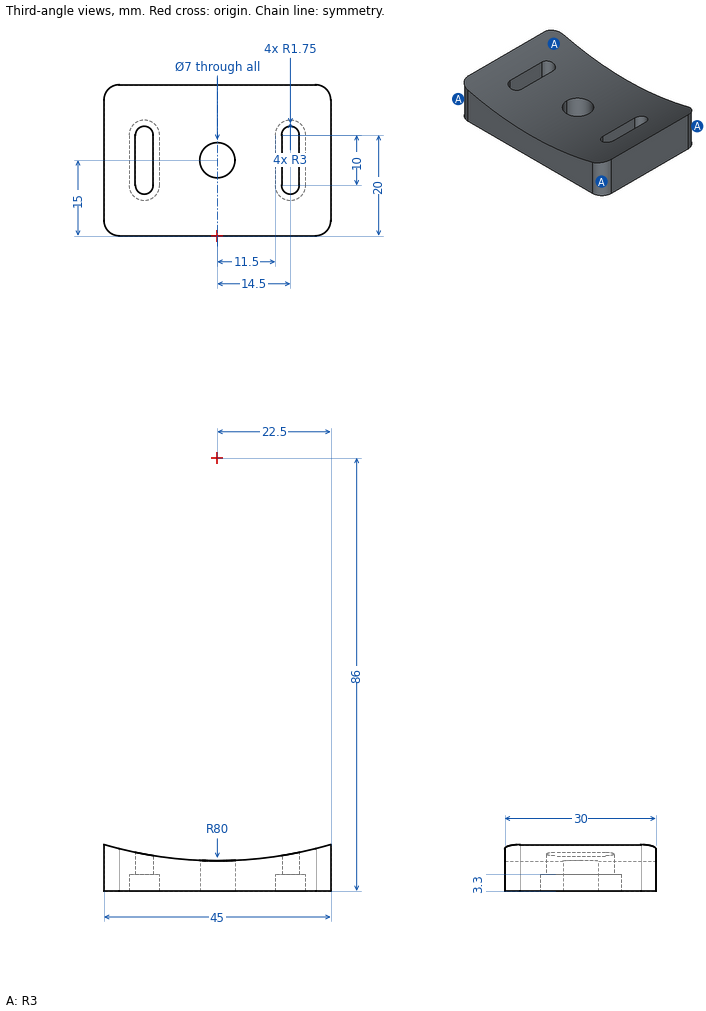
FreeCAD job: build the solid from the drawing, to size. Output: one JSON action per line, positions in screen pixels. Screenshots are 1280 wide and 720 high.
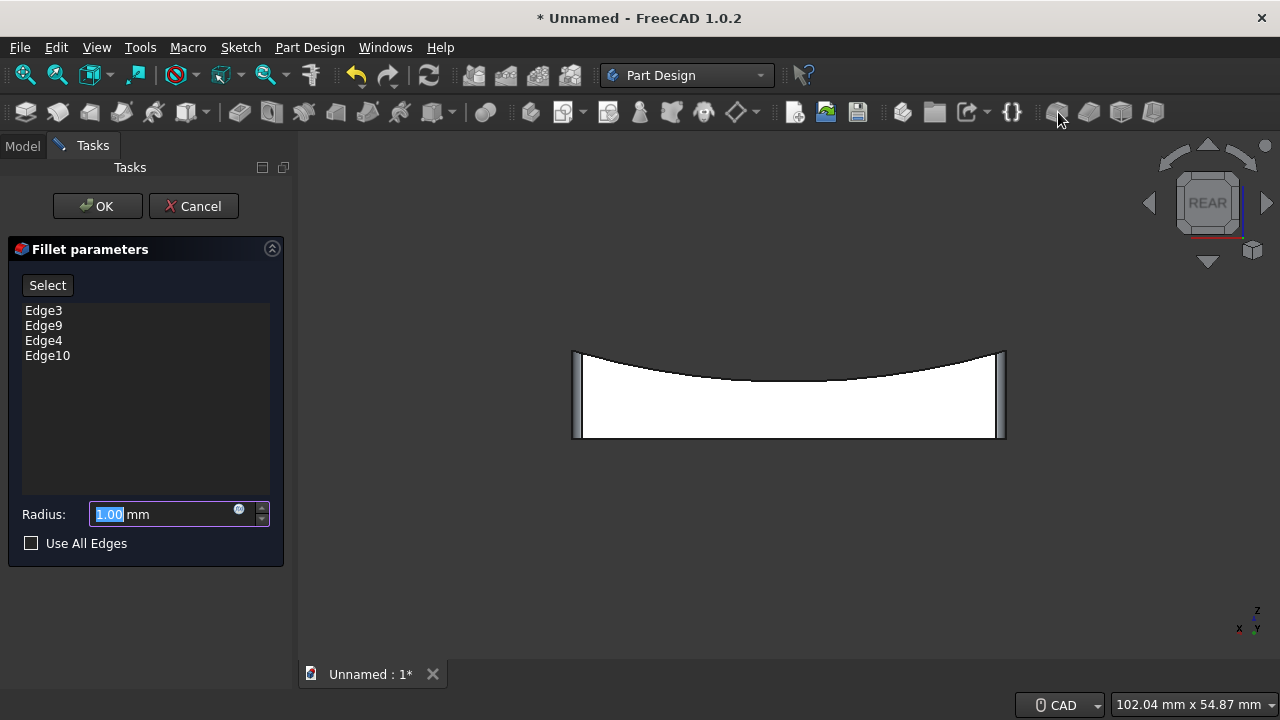
{"action": "type", "text": "3"}
{"action": "key", "text": "Tab"}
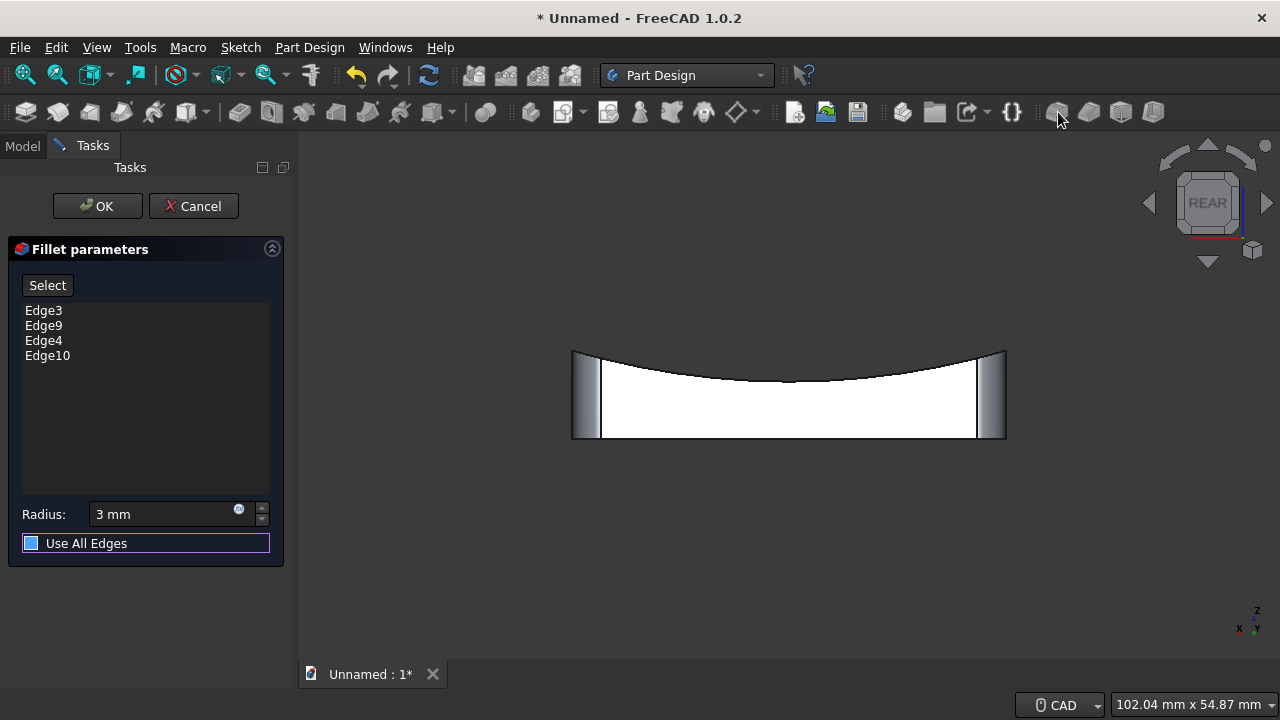
{"action": "left_click", "coordinate": [98, 206]}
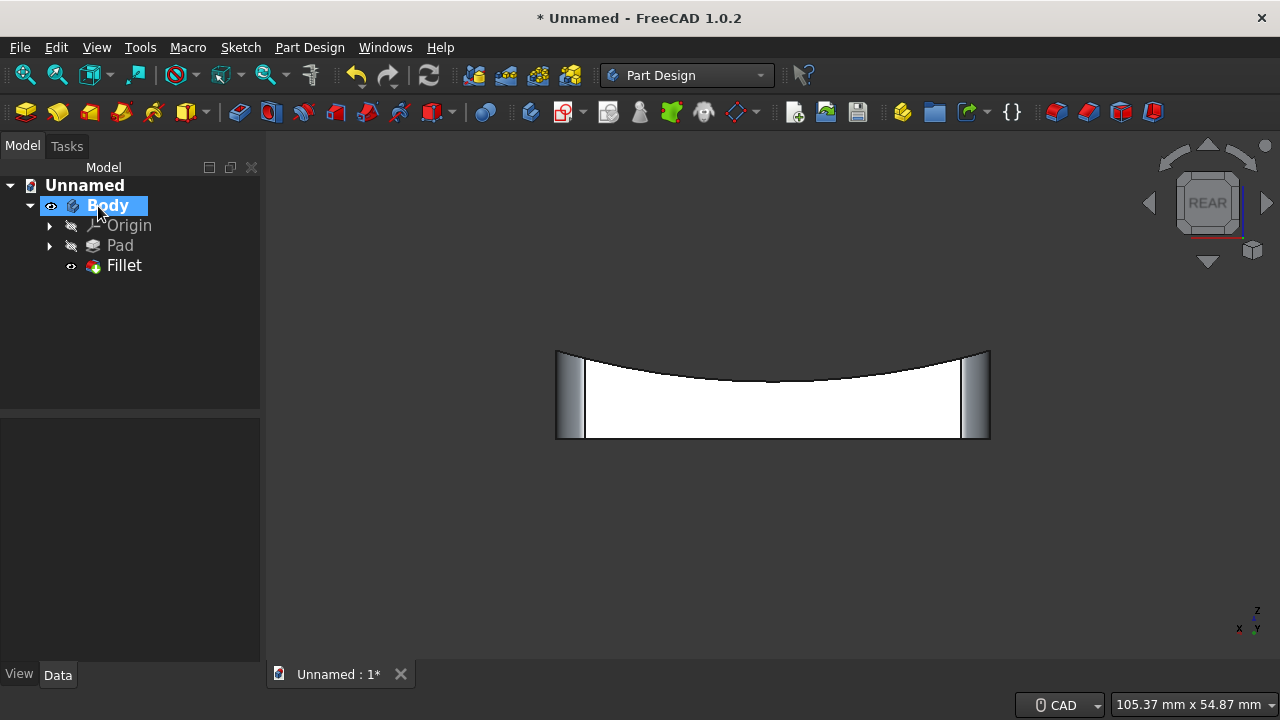
{"action": "key", "text": "v f"}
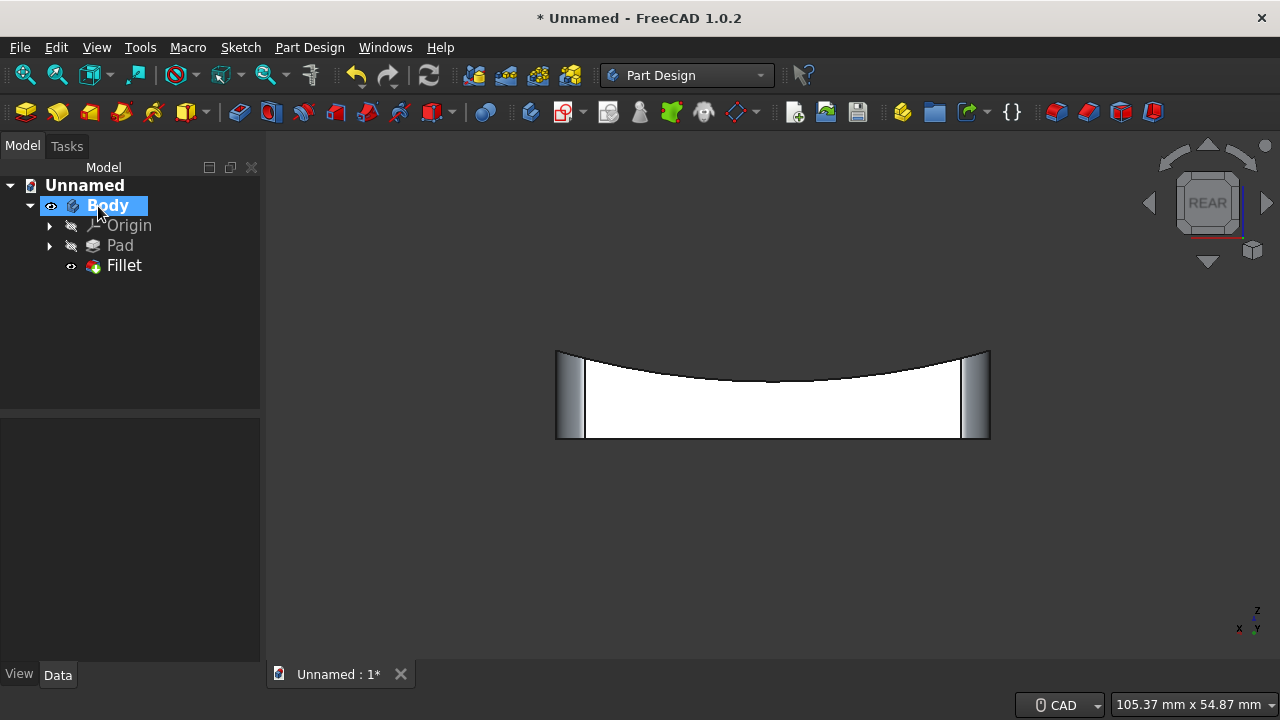
{"action": "key", "text": "5"}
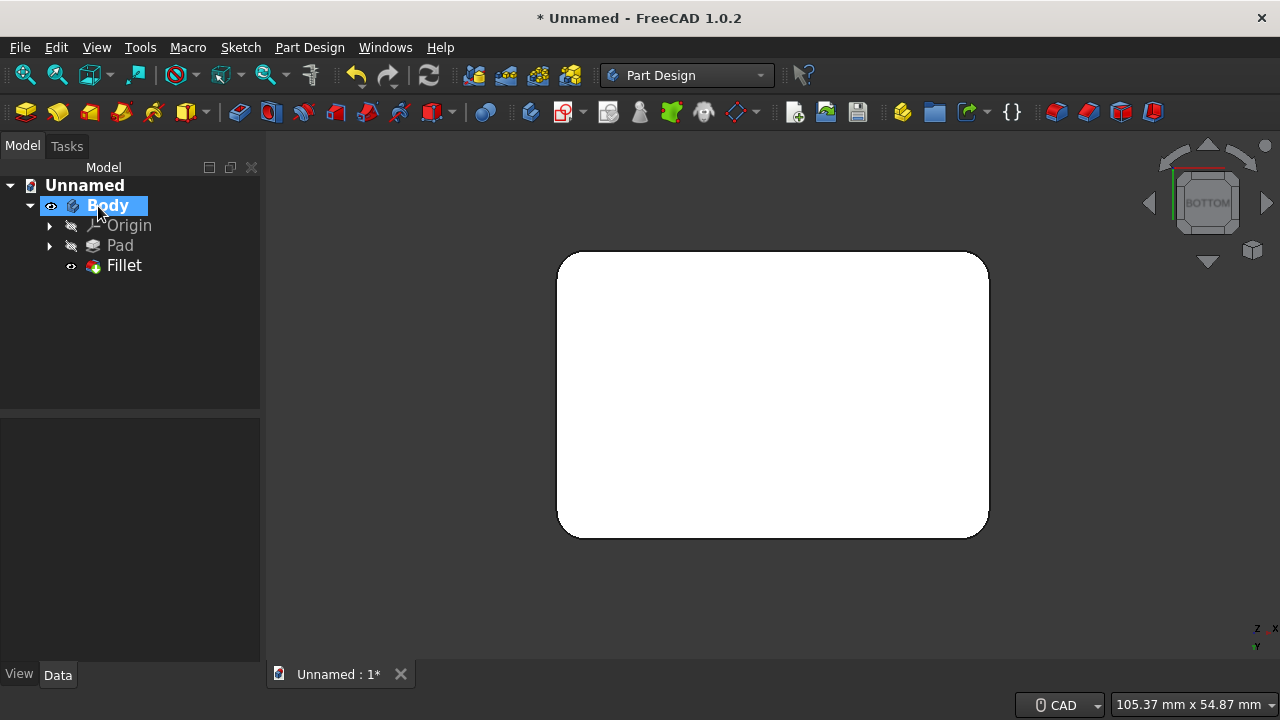
{"action": "left_click", "coordinate": [835, 394]}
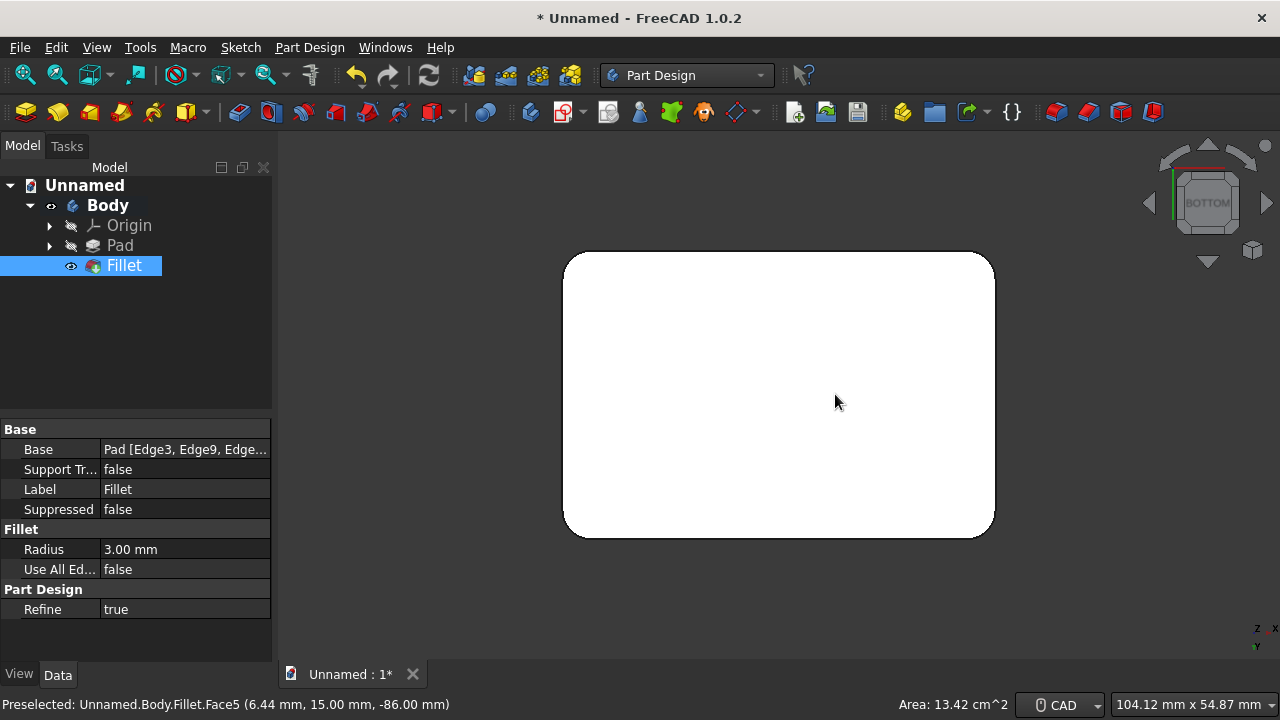
{"action": "left_click", "coordinate": [564, 112]}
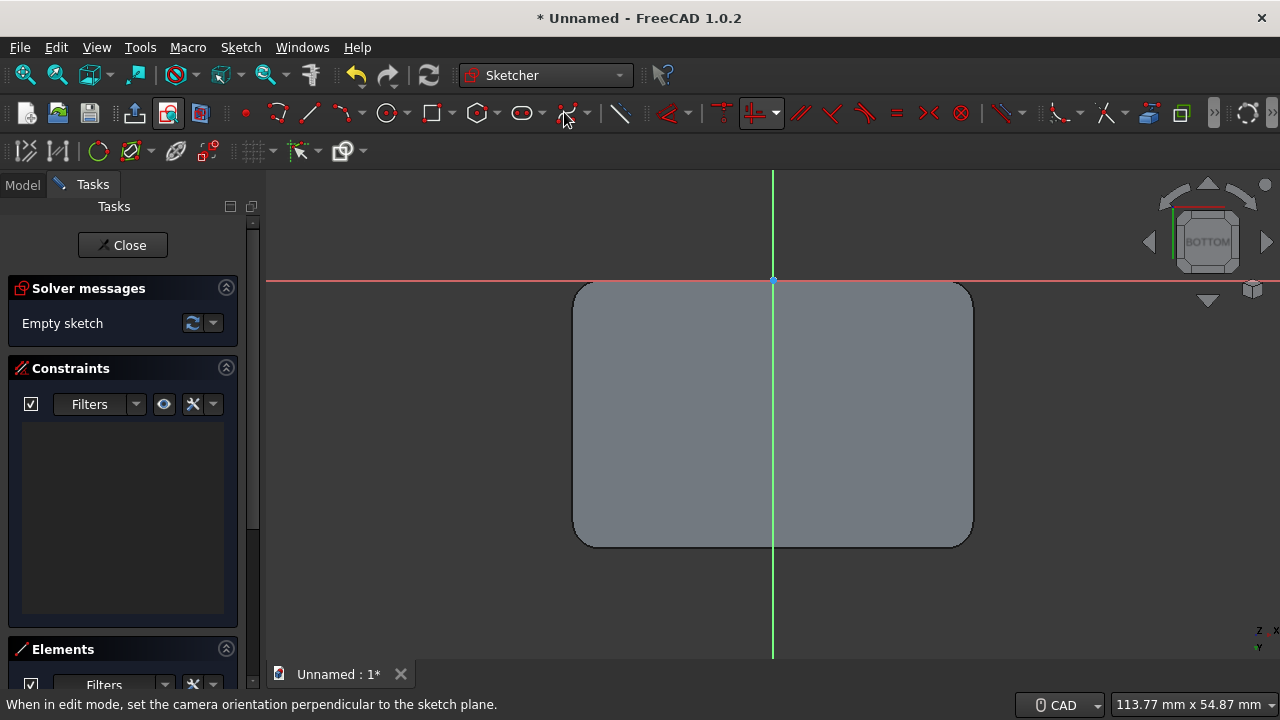
{"action": "scroll", "coordinate": [790, 414], "scroll_direction": "up", "scroll_amount": 8}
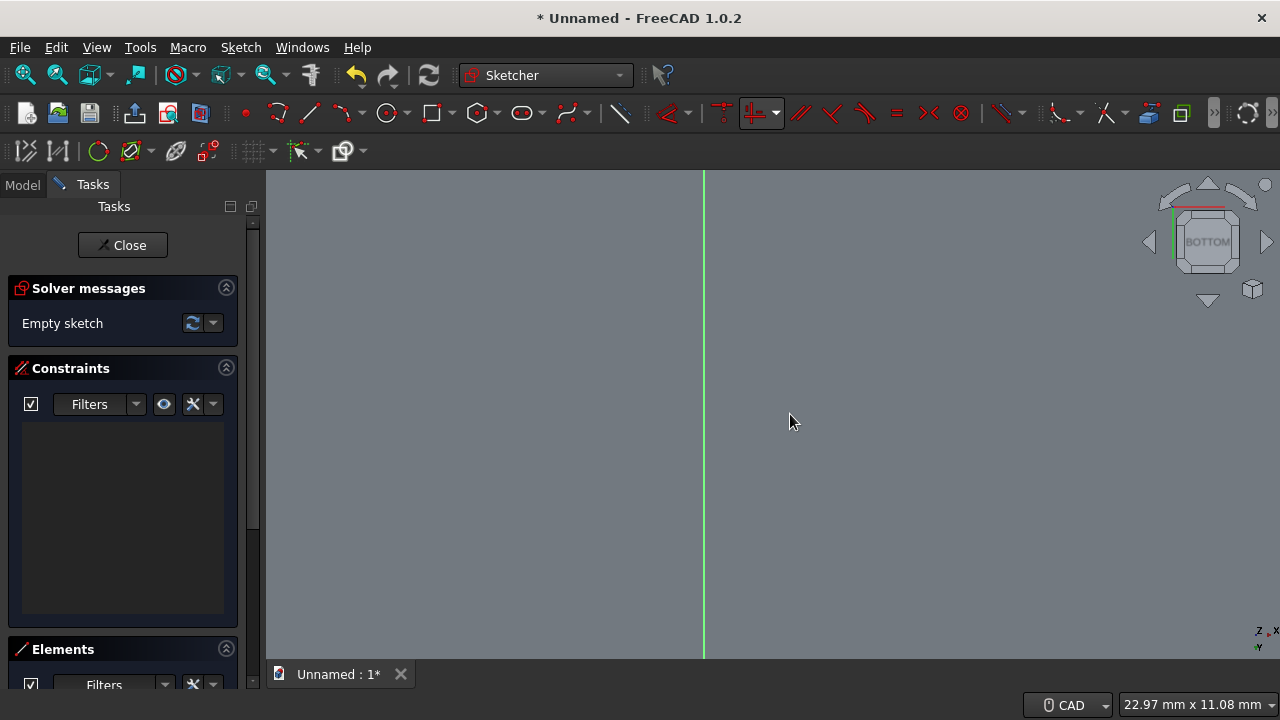
{"action": "left_click", "coordinate": [388, 114]}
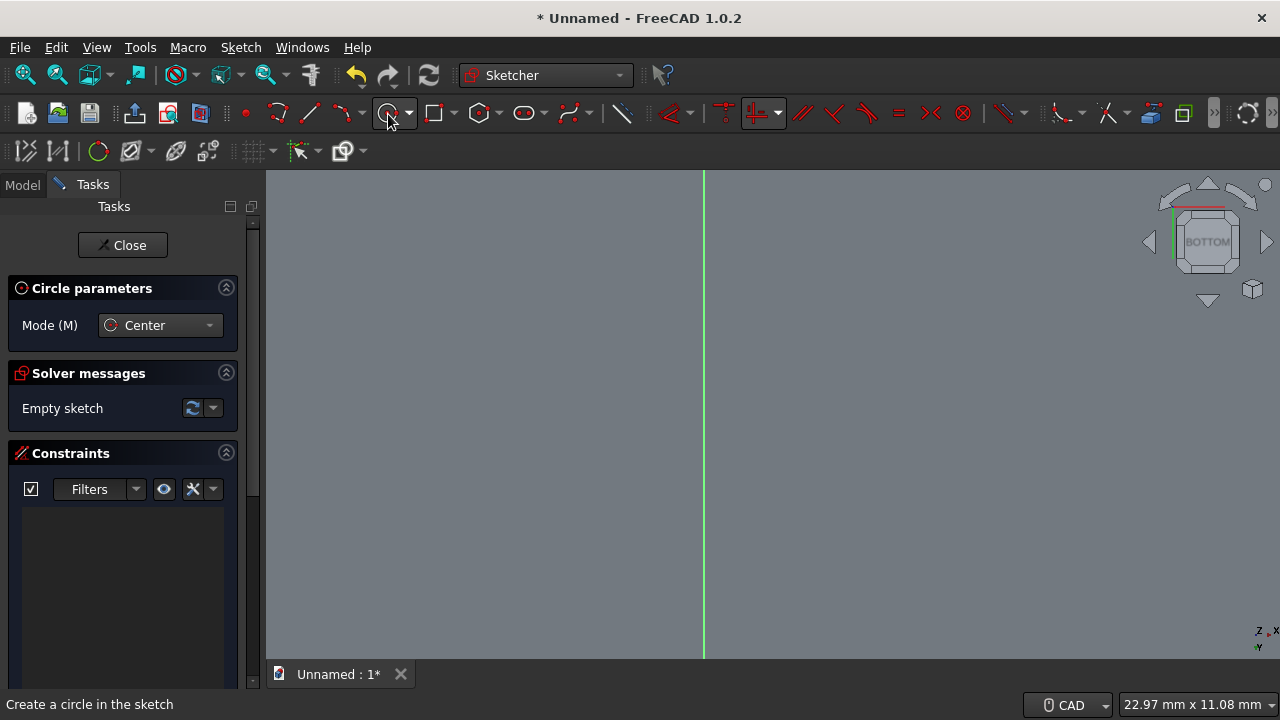
{"action": "left_click", "coordinate": [704, 414]}
{"action": "mouse_move", "coordinate": [813, 305]}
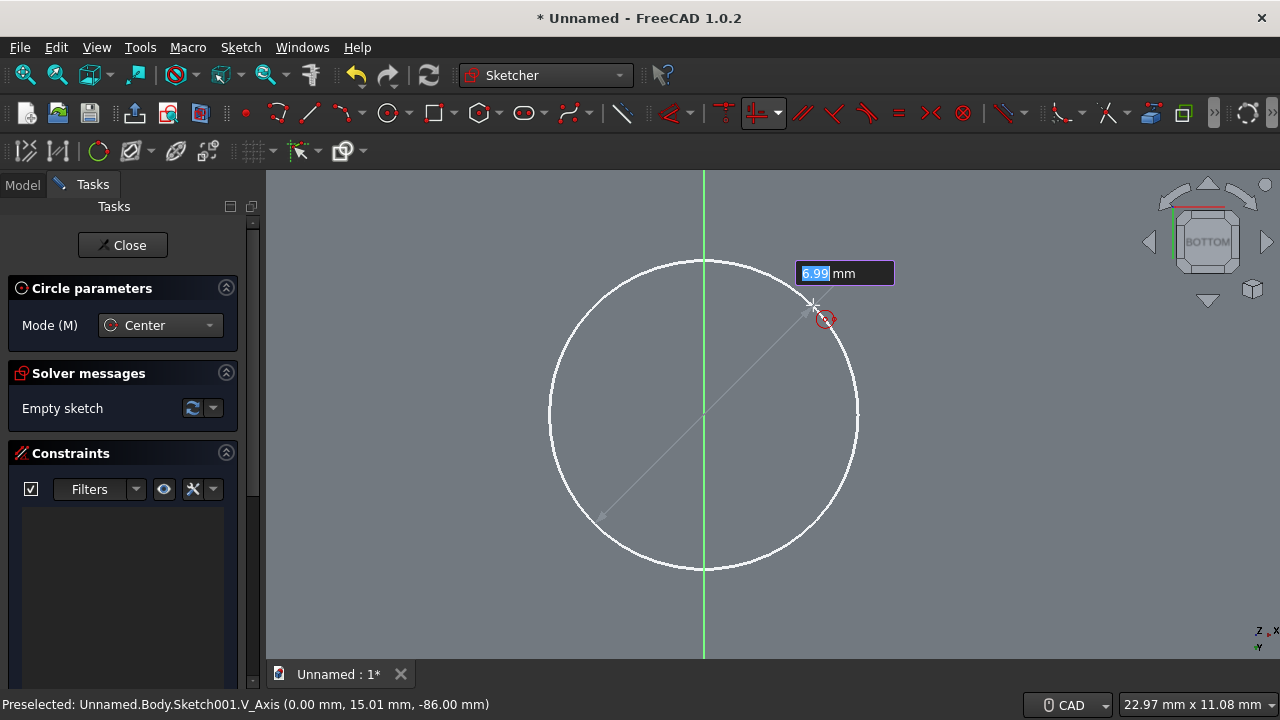
{"action": "type", "text": "7"}
{"action": "key", "text": "Return"}
{"action": "key", "text": "Escape"}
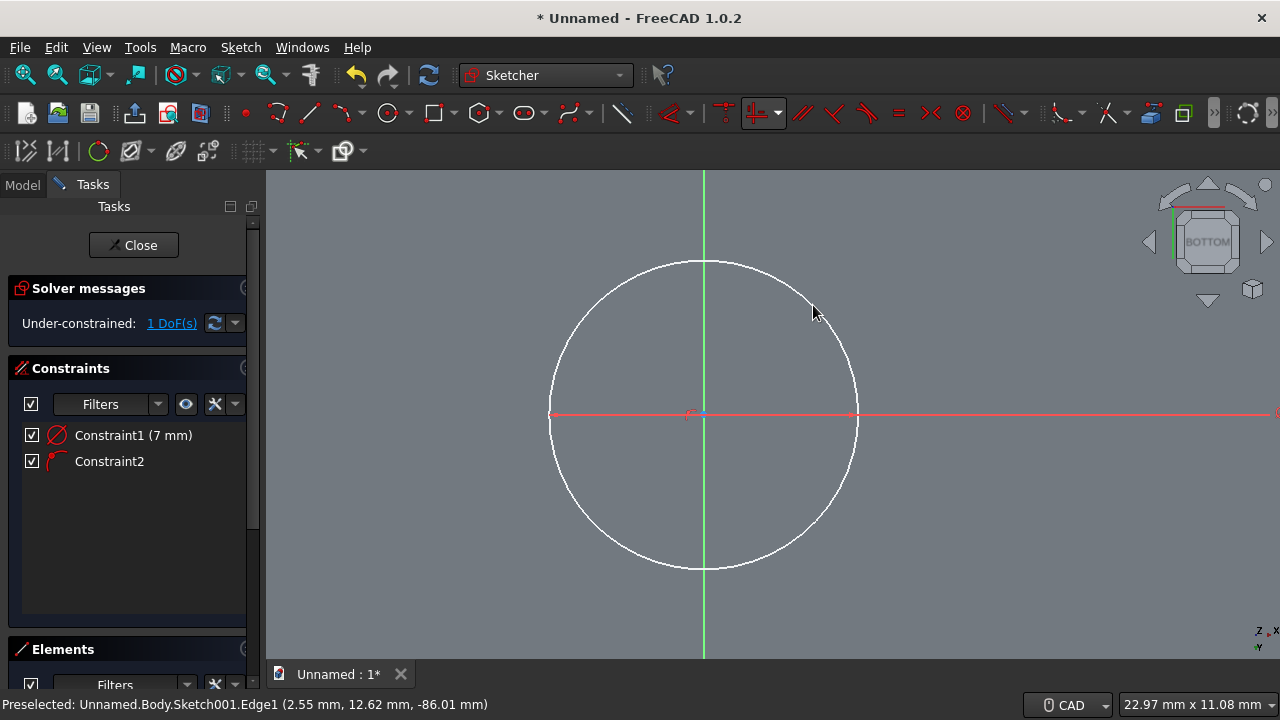
{"action": "left_click", "coordinate": [670, 114]}